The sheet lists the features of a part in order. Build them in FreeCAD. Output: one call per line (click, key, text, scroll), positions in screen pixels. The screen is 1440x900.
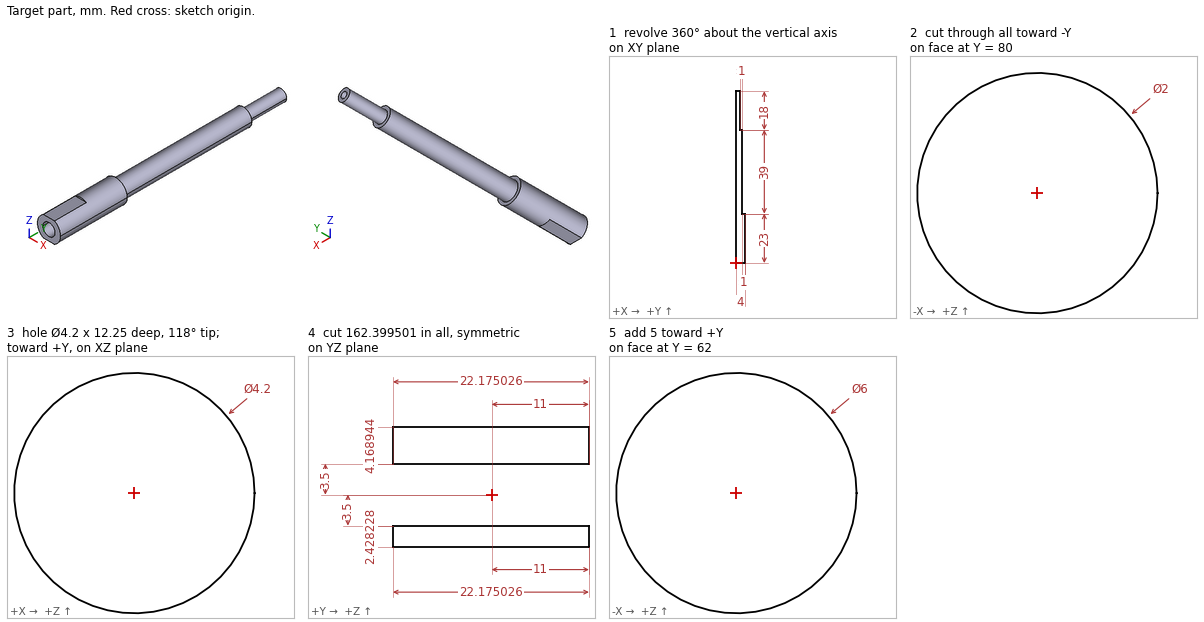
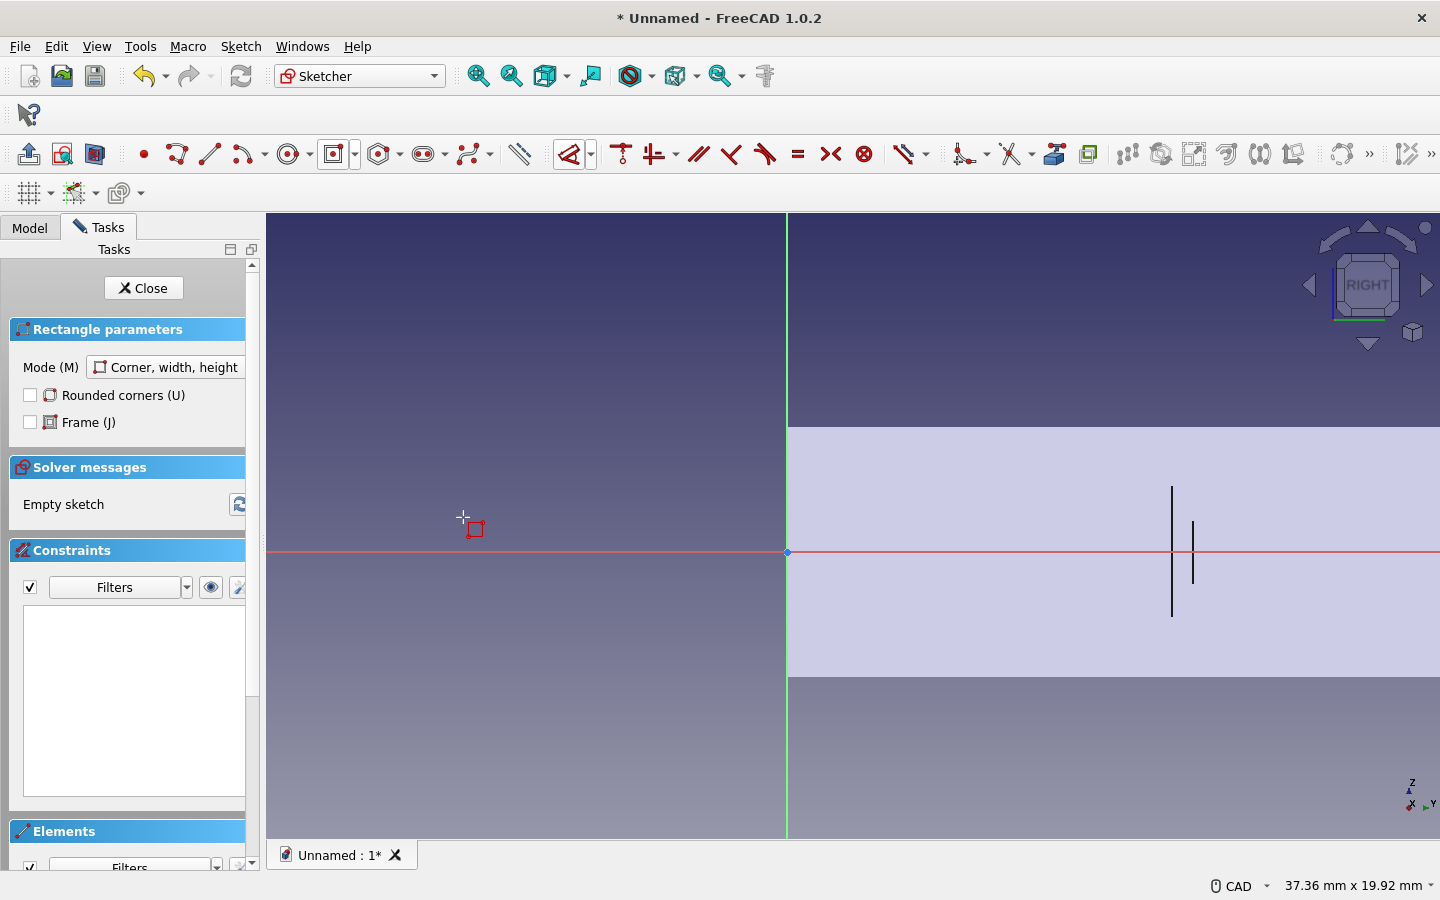
click(436, 311)
click(1133, 442)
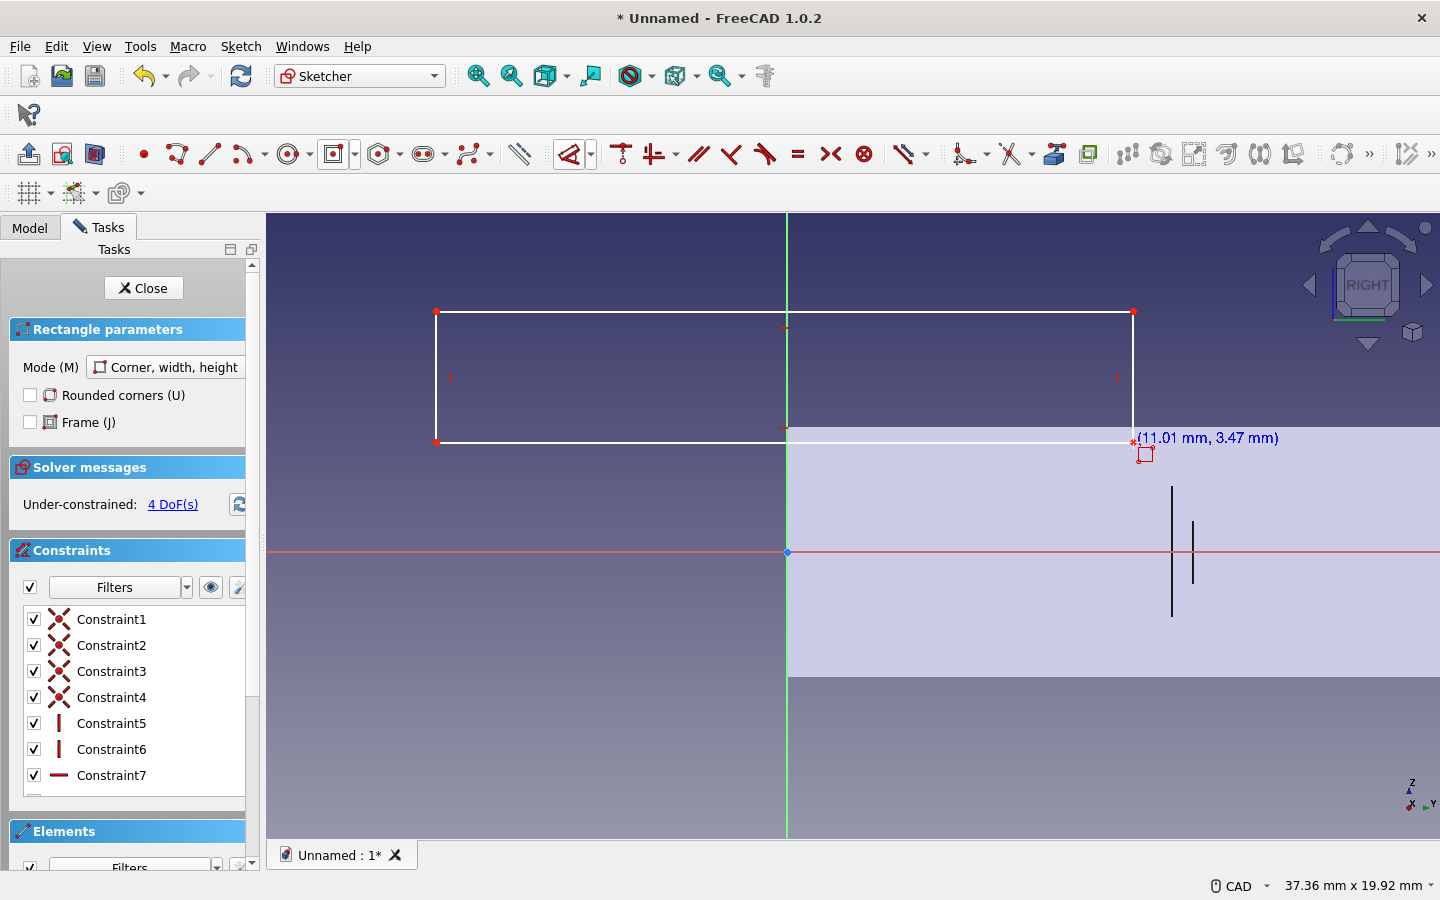
click(436, 662)
click(1133, 738)
key(Escape)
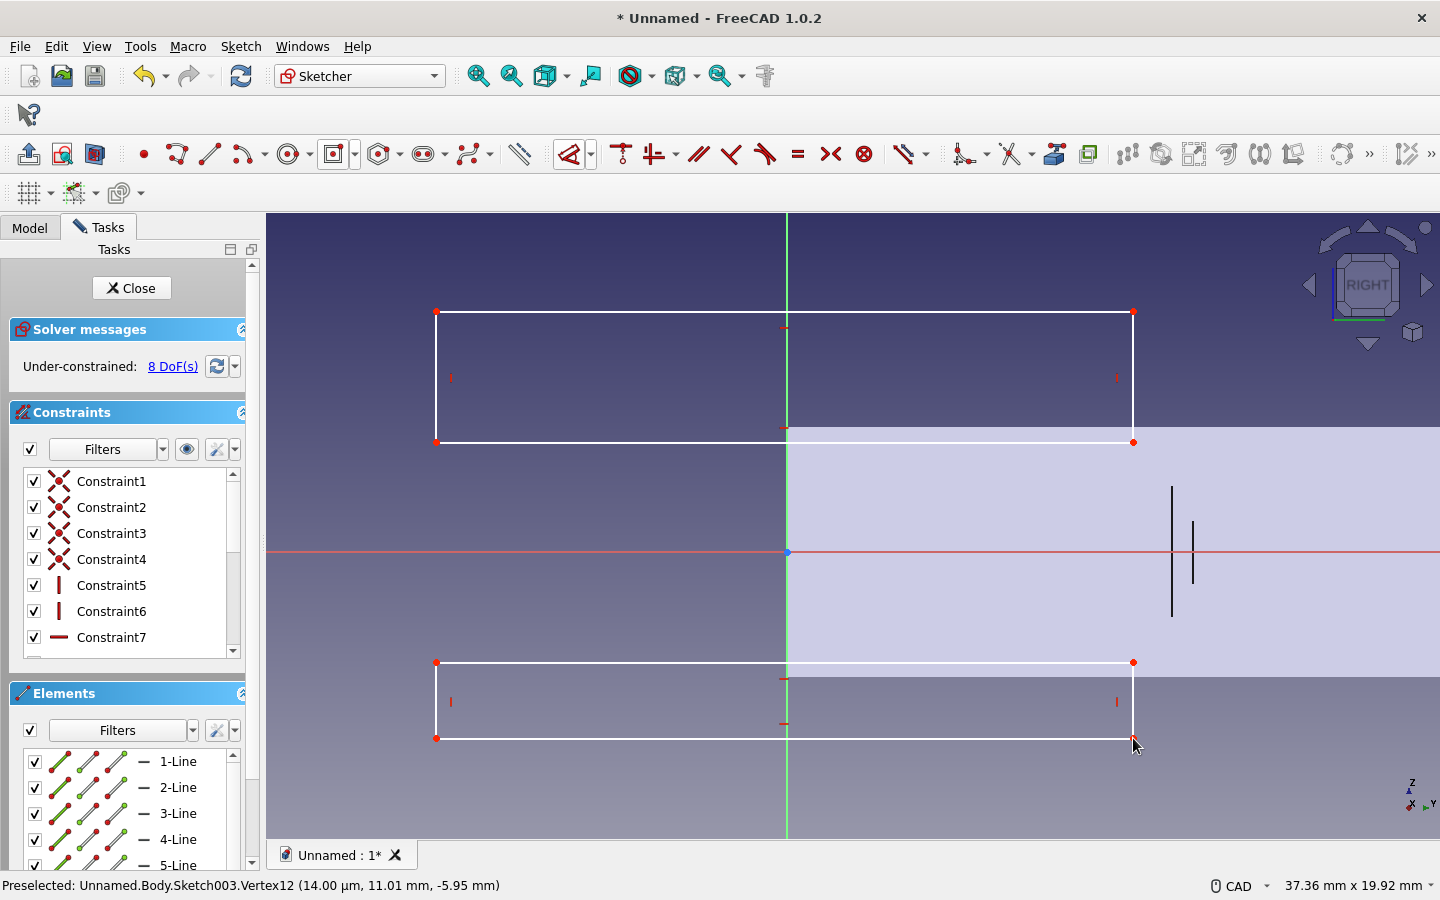
click(1133, 443)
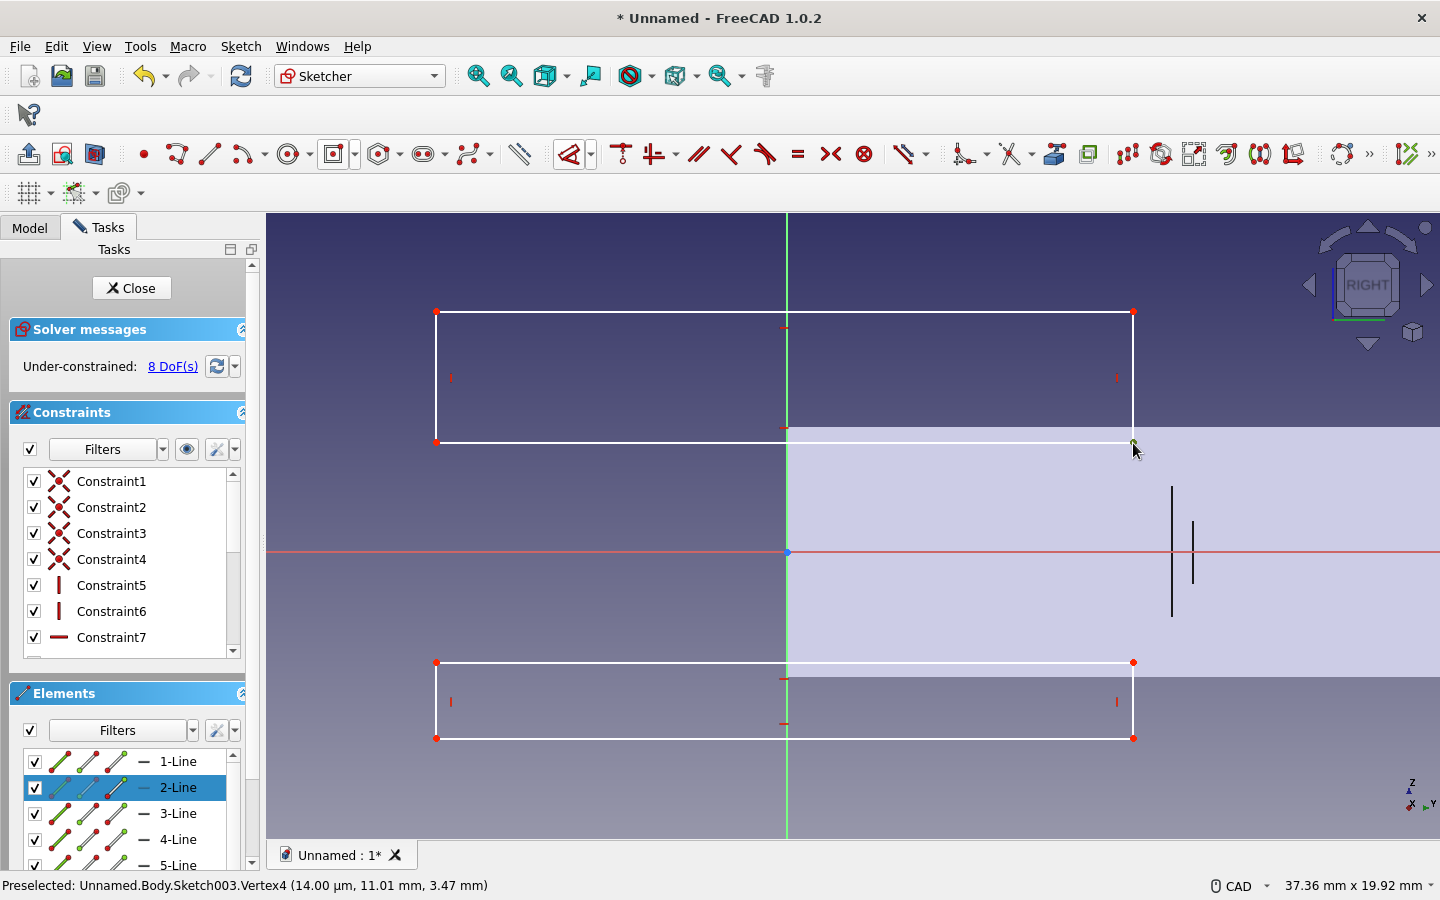
key(l)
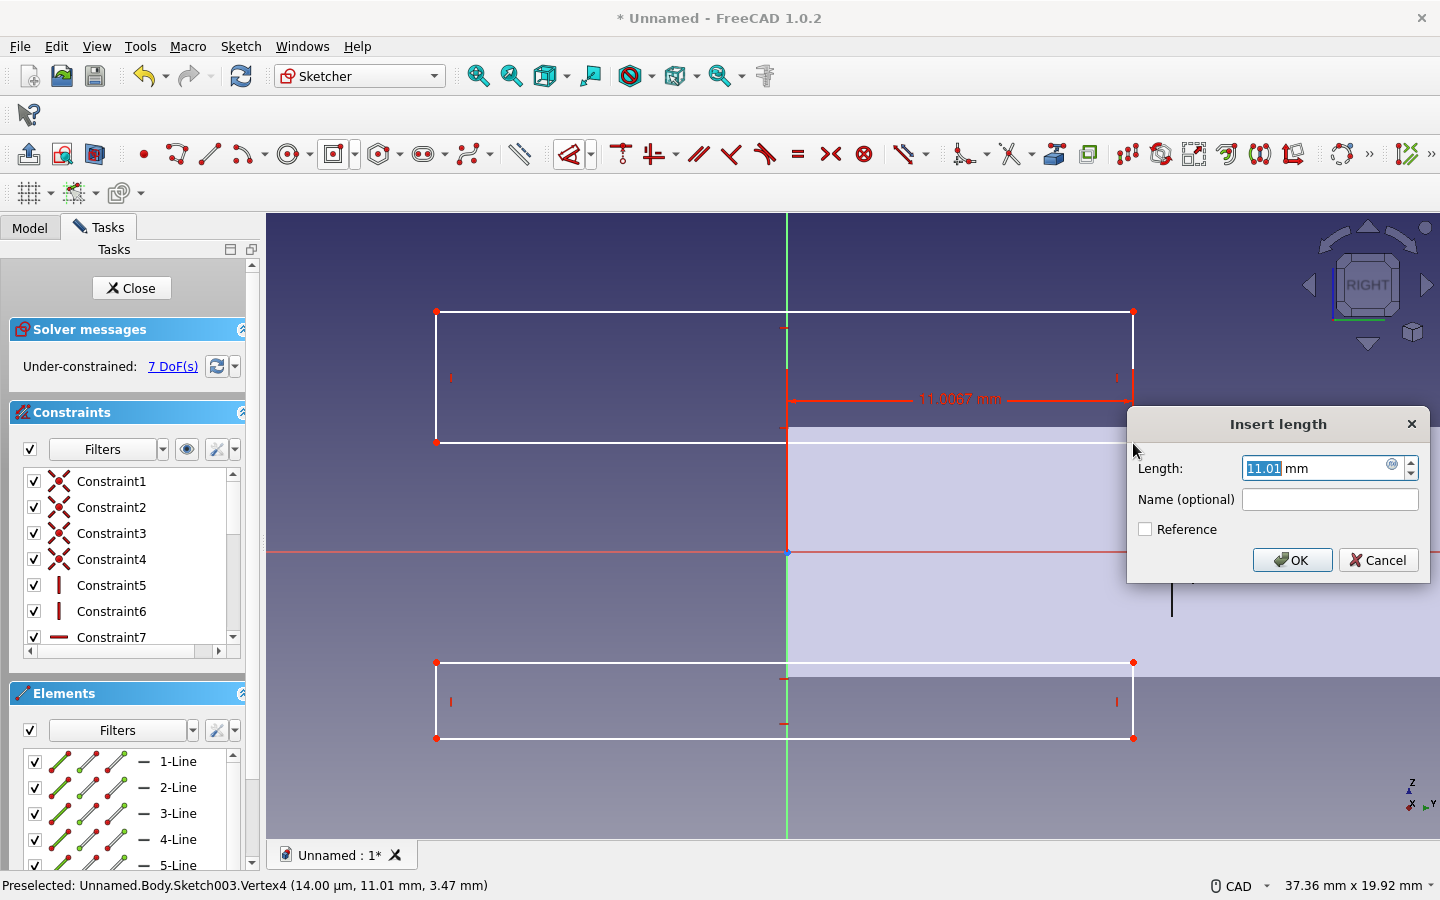
text(11)
key(Return)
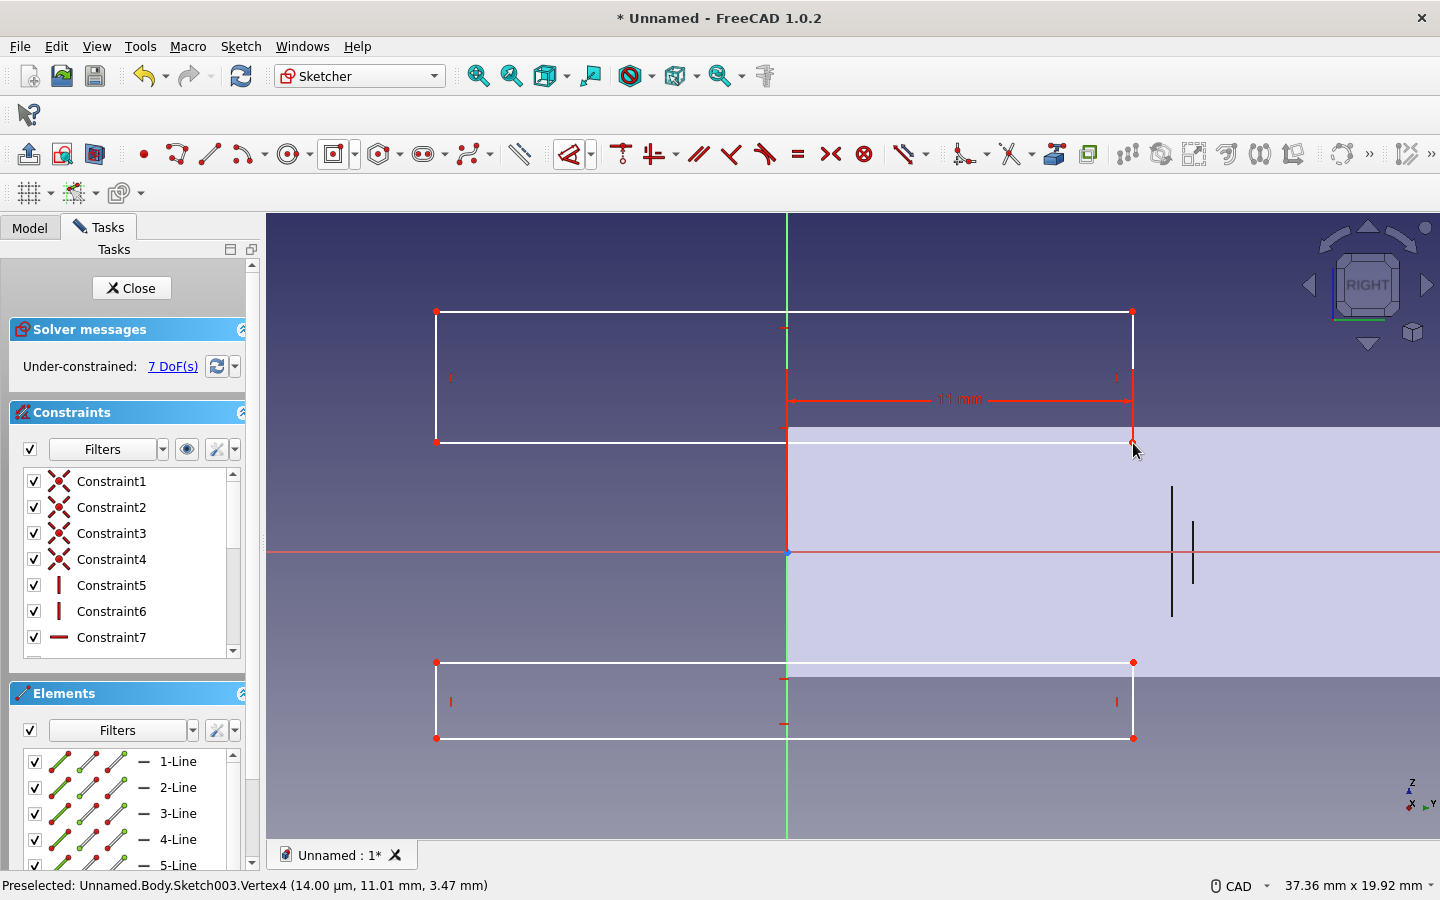
click(1133, 739)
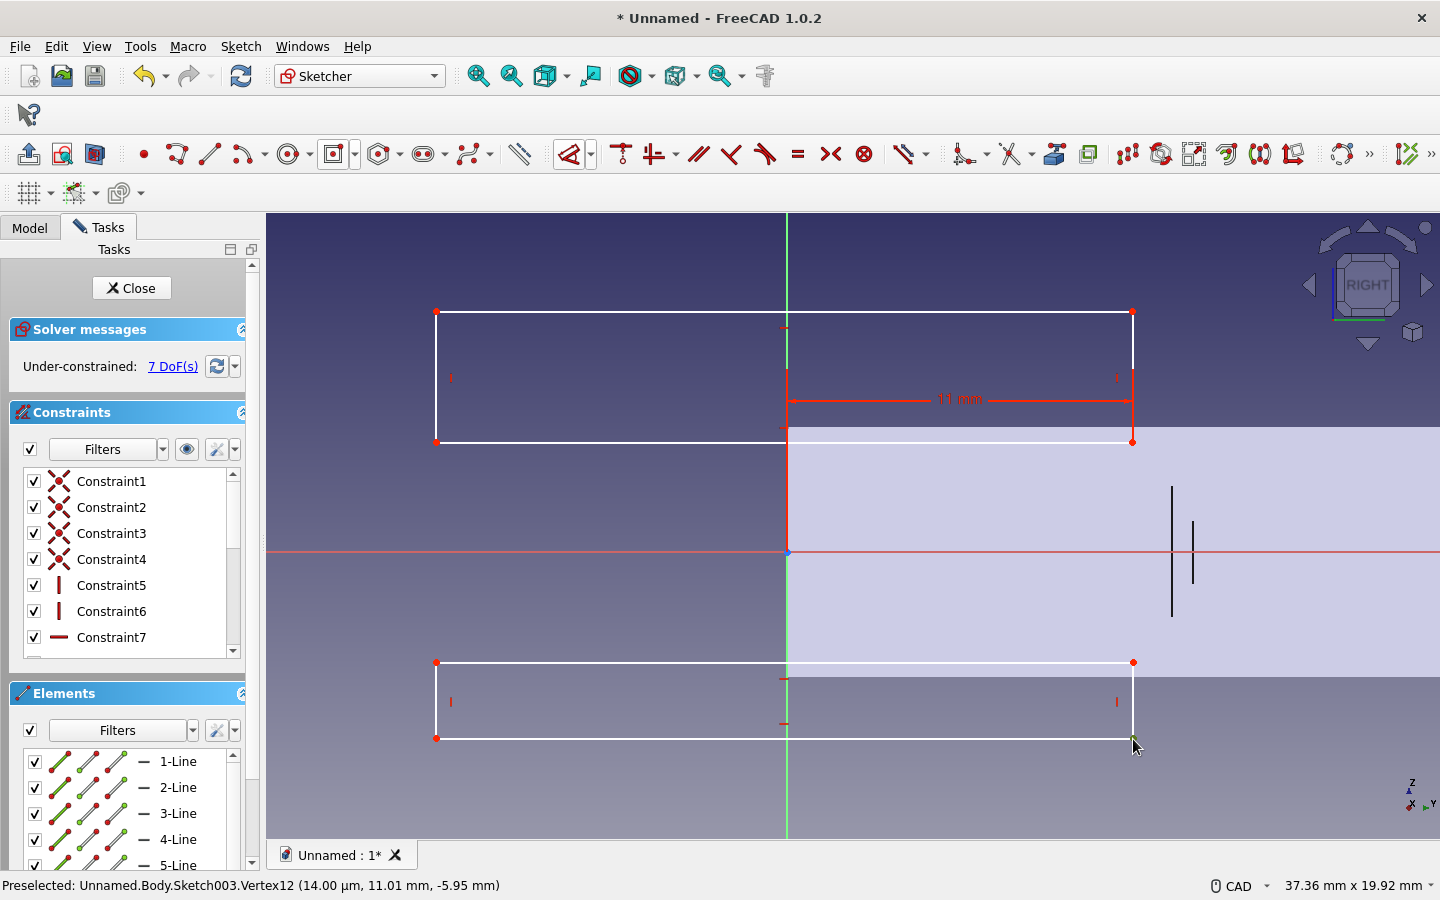
key(l)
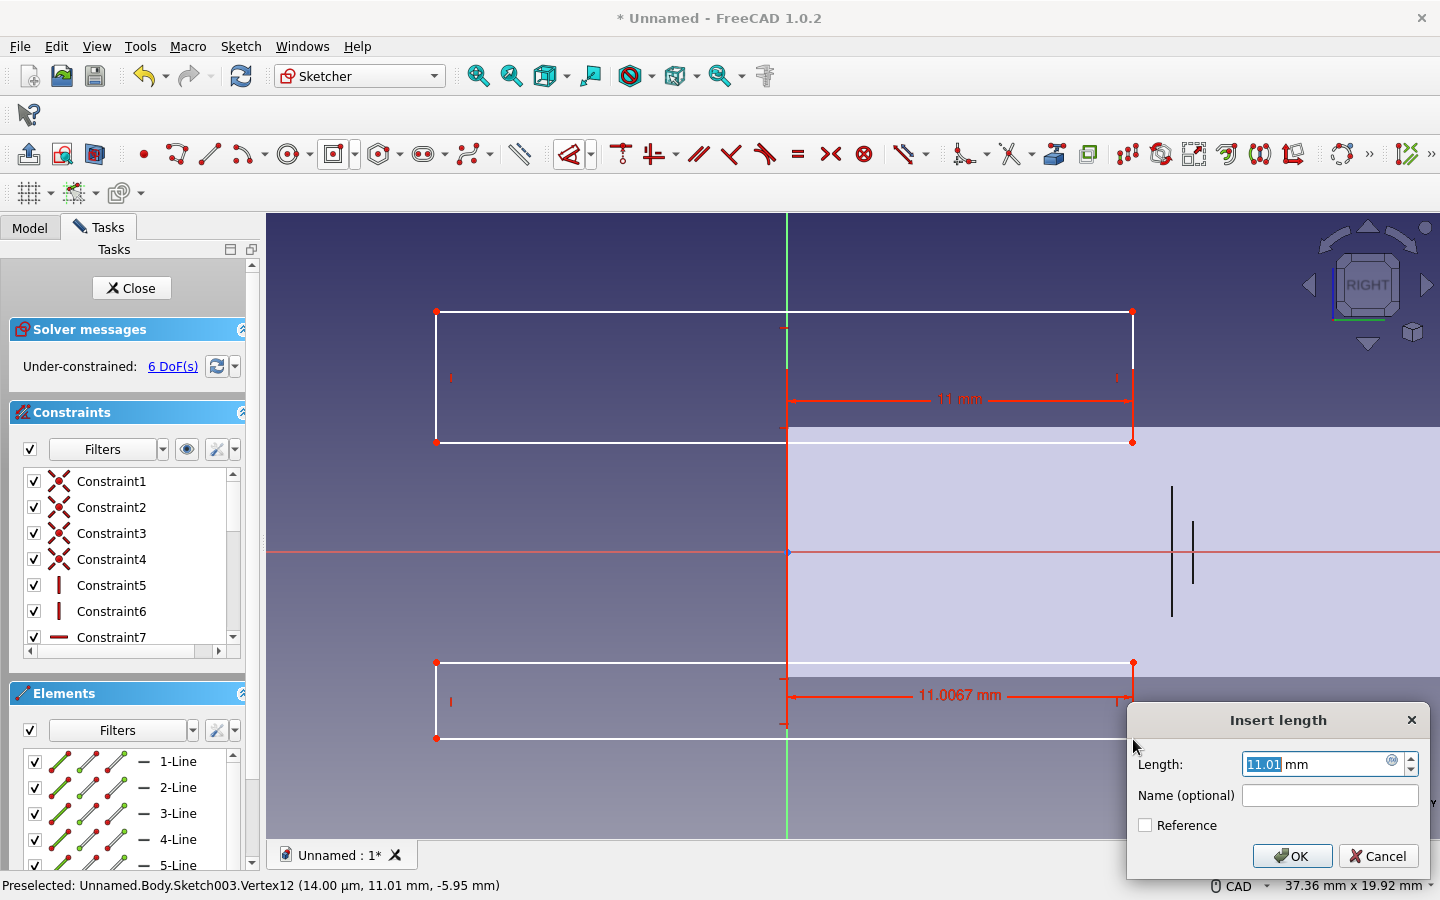
text(11)
key(Return)